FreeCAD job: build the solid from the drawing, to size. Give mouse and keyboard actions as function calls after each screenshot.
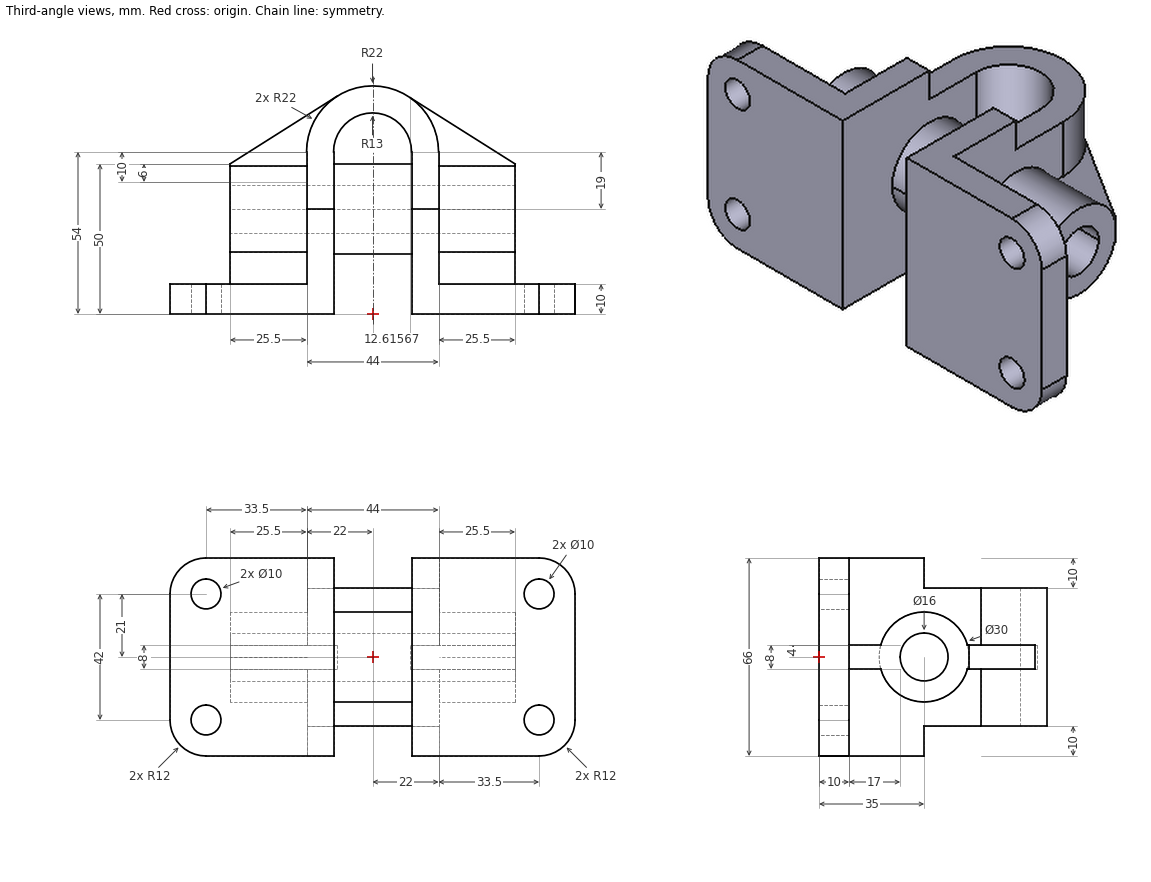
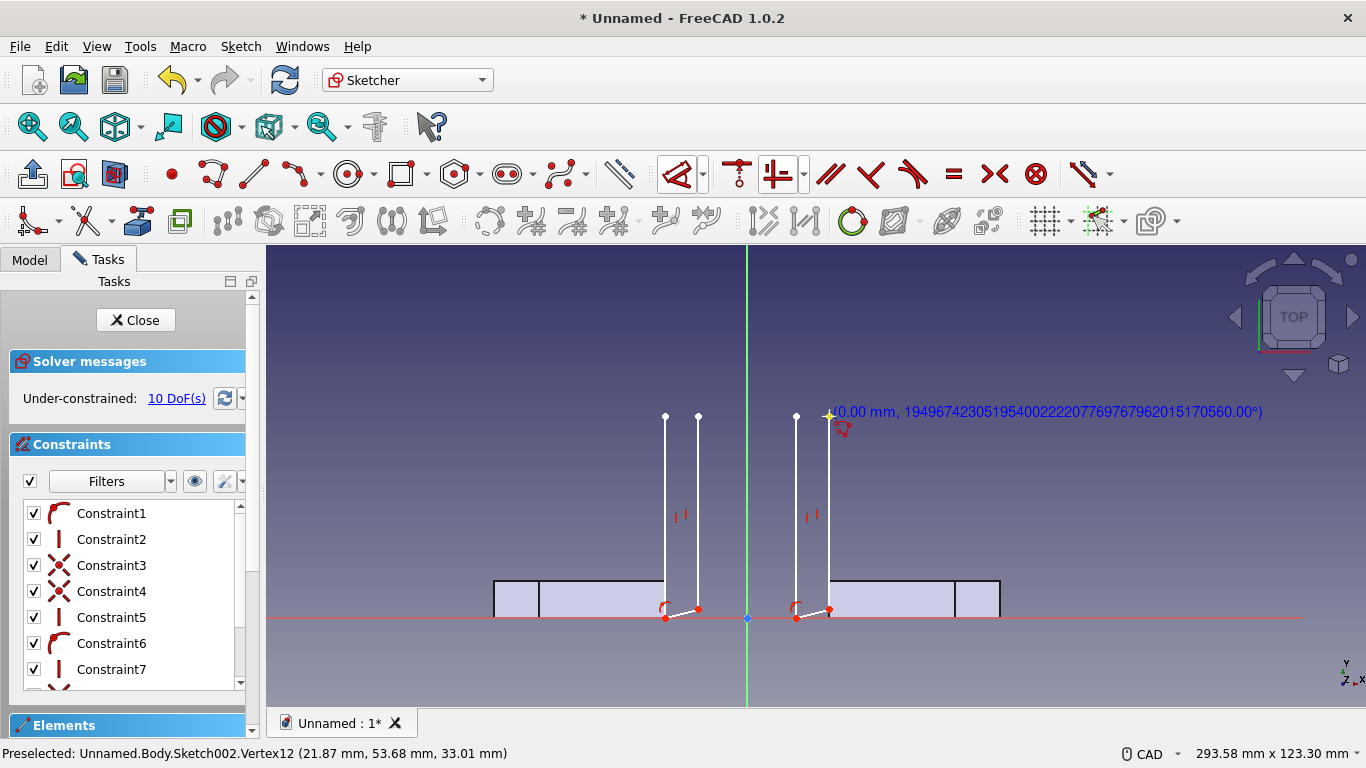
click(294, 174)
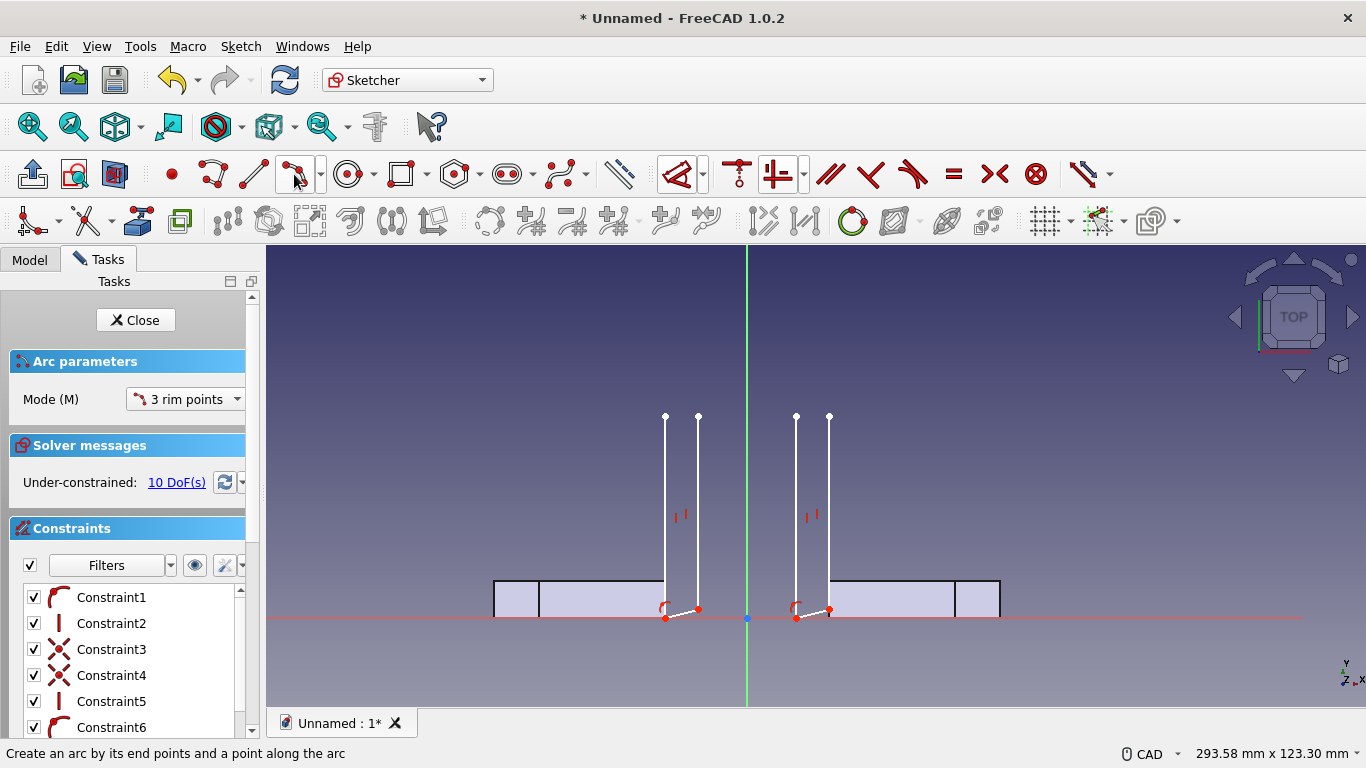
click(698, 417)
click(796, 417)
click(762, 369)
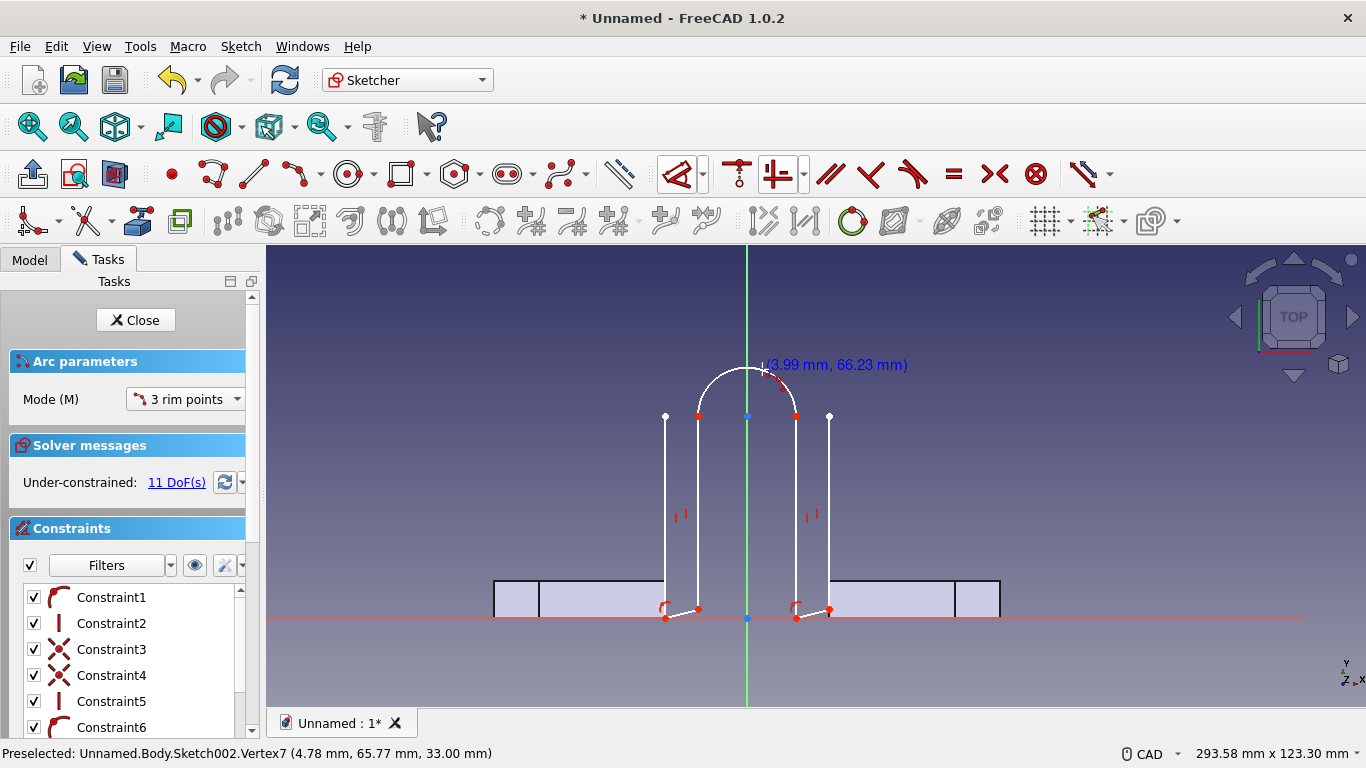
click(829, 417)
click(665, 417)
click(773, 337)
key(Escape)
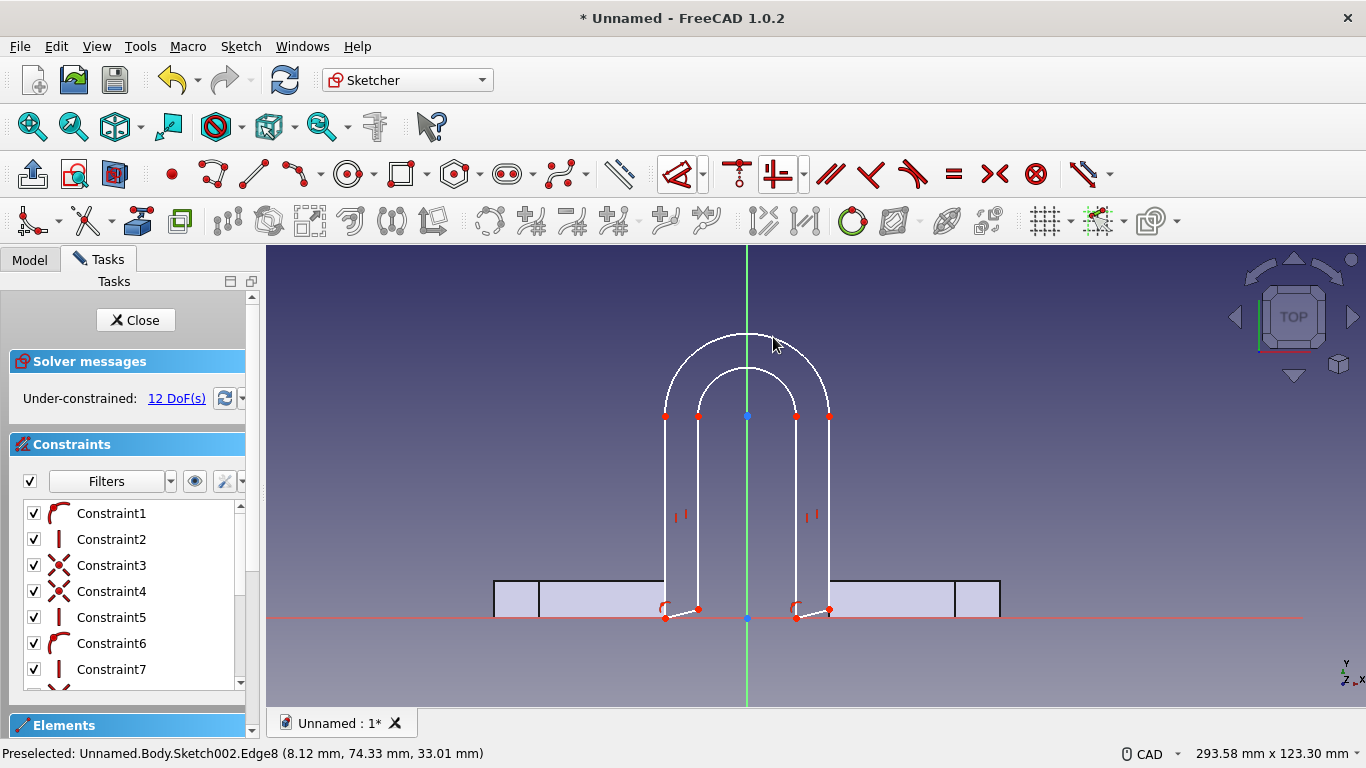
click(665, 477)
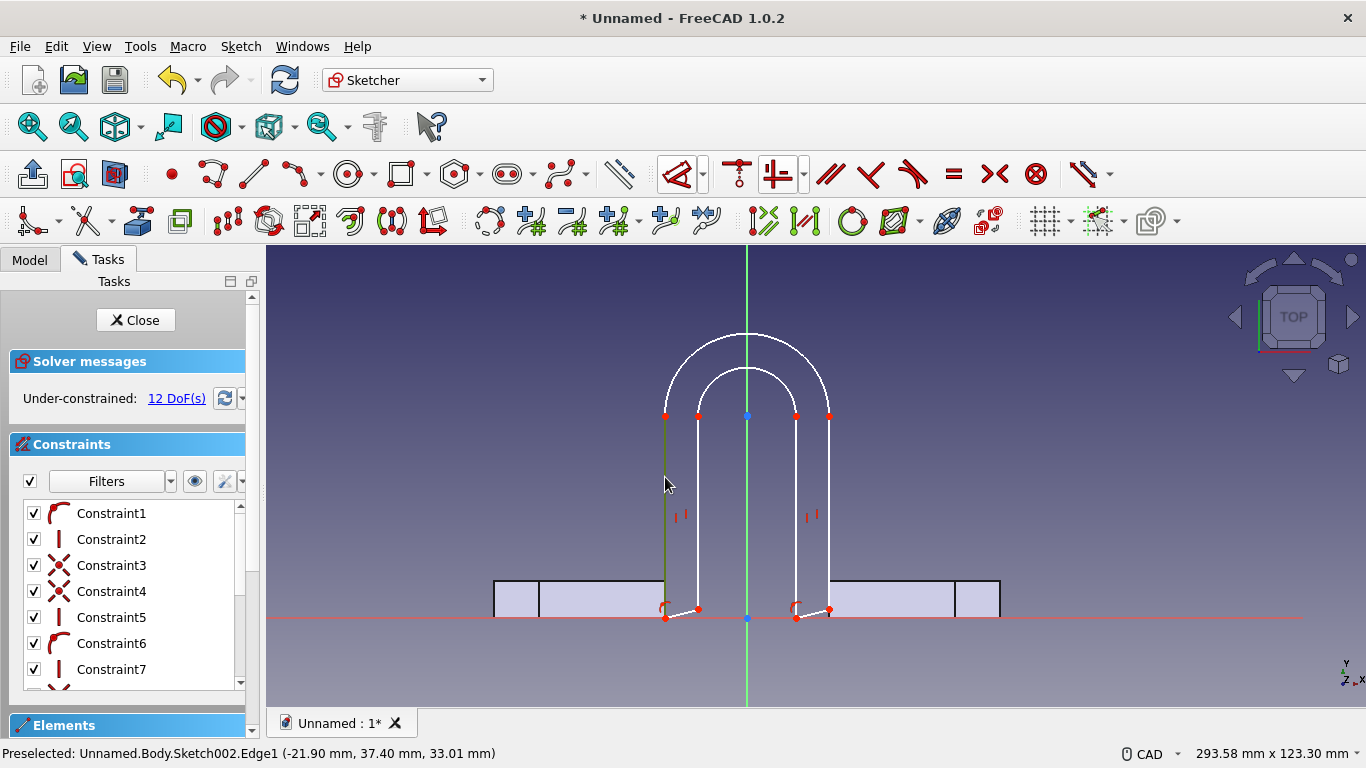
click(796, 350)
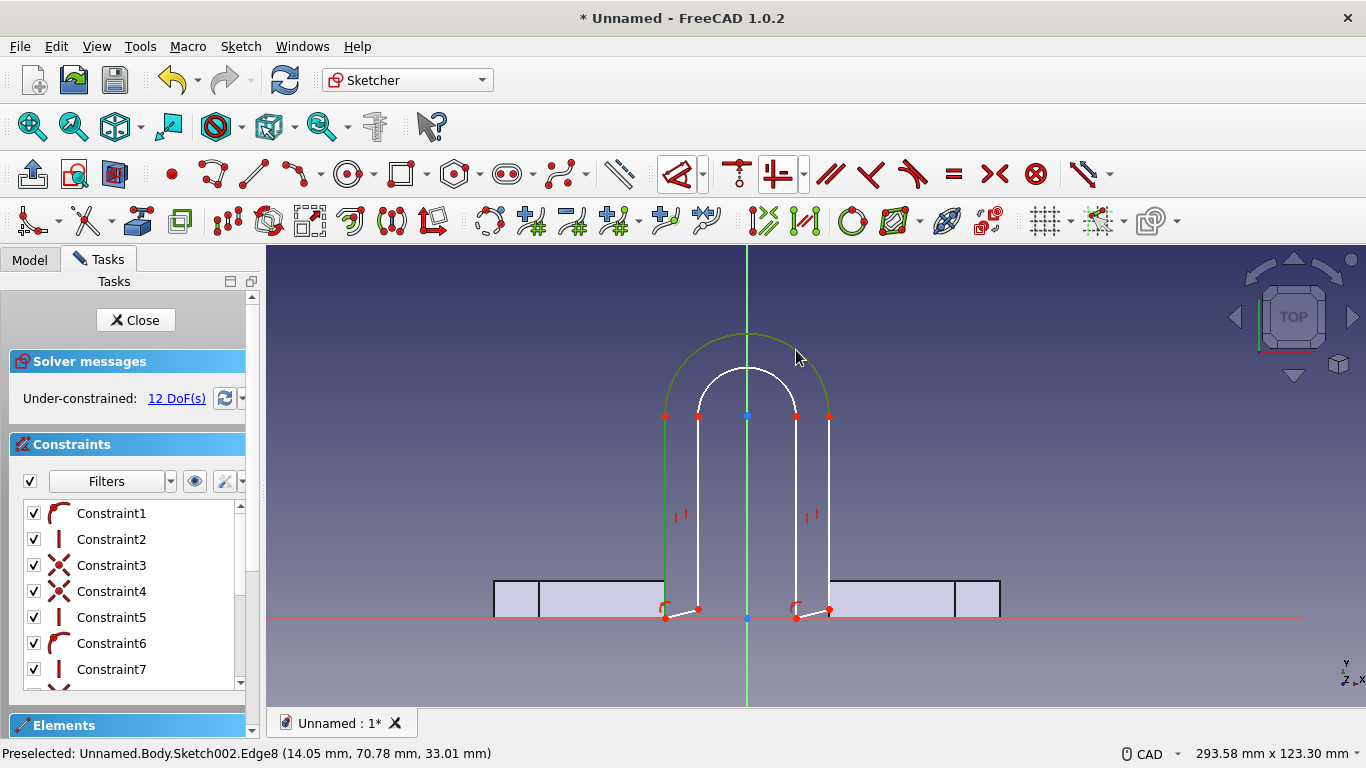
click(913, 174)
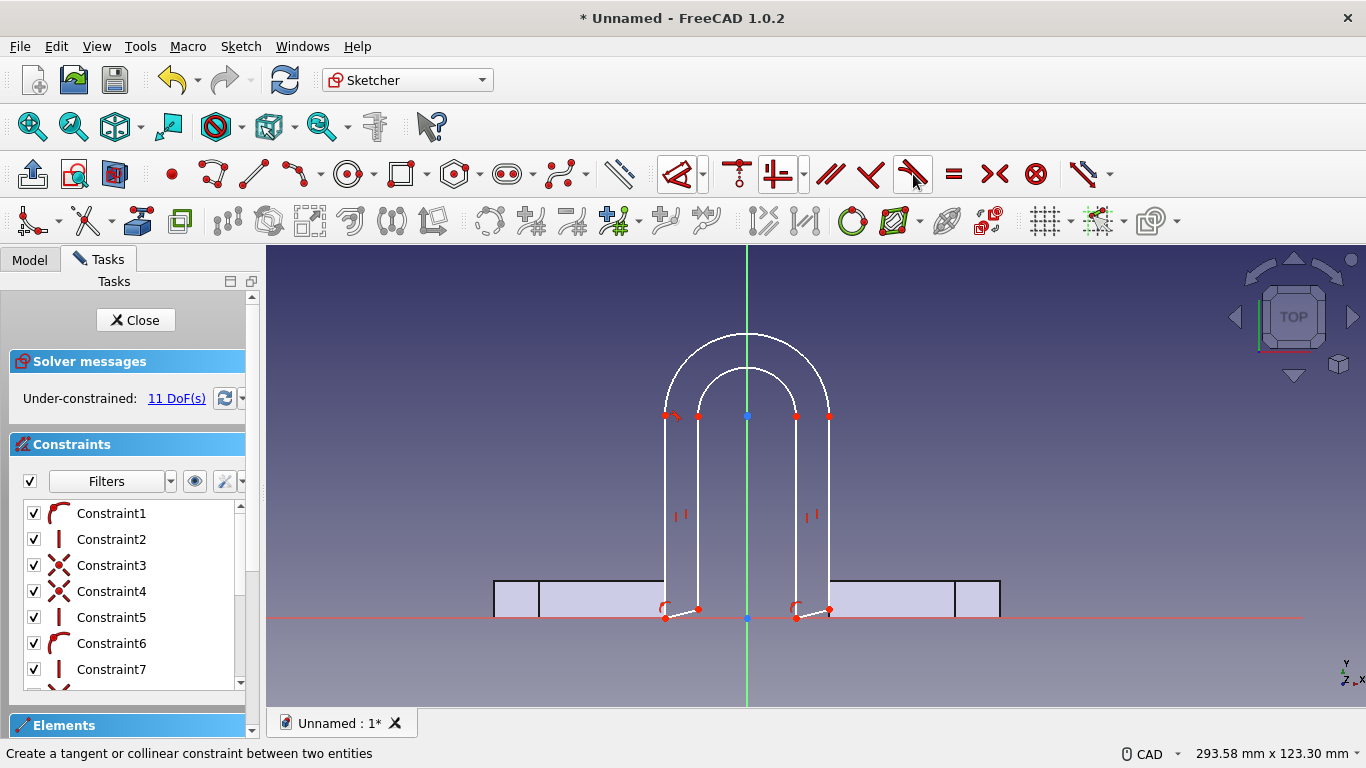
click(698, 552)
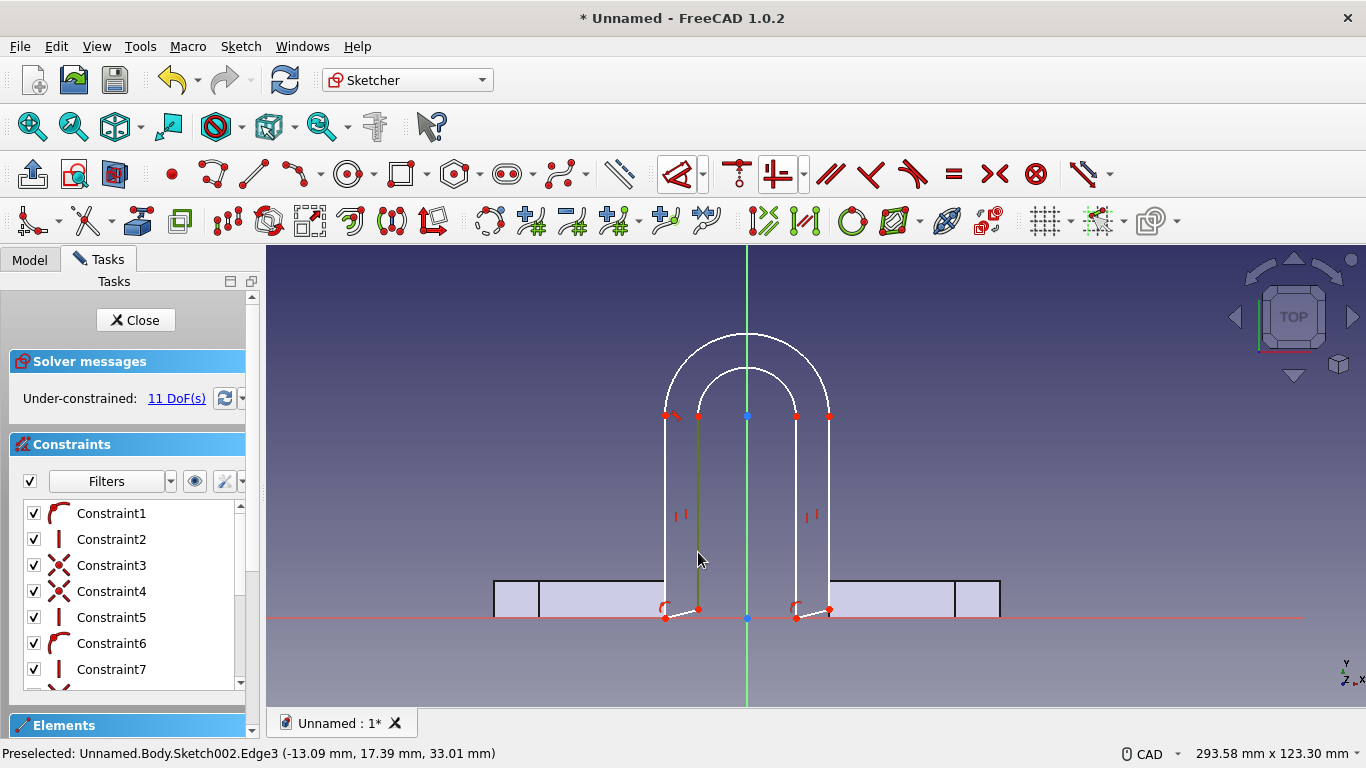
click(776, 377)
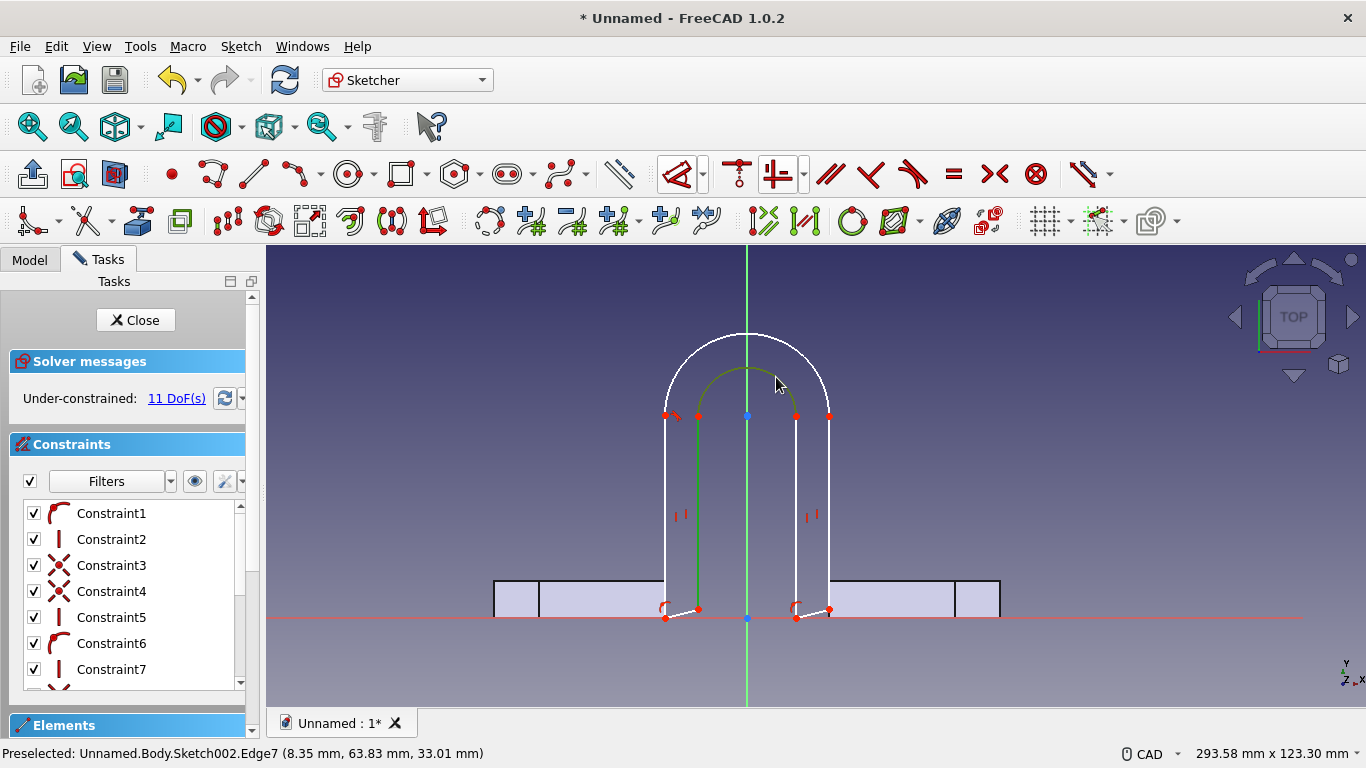
click(913, 174)